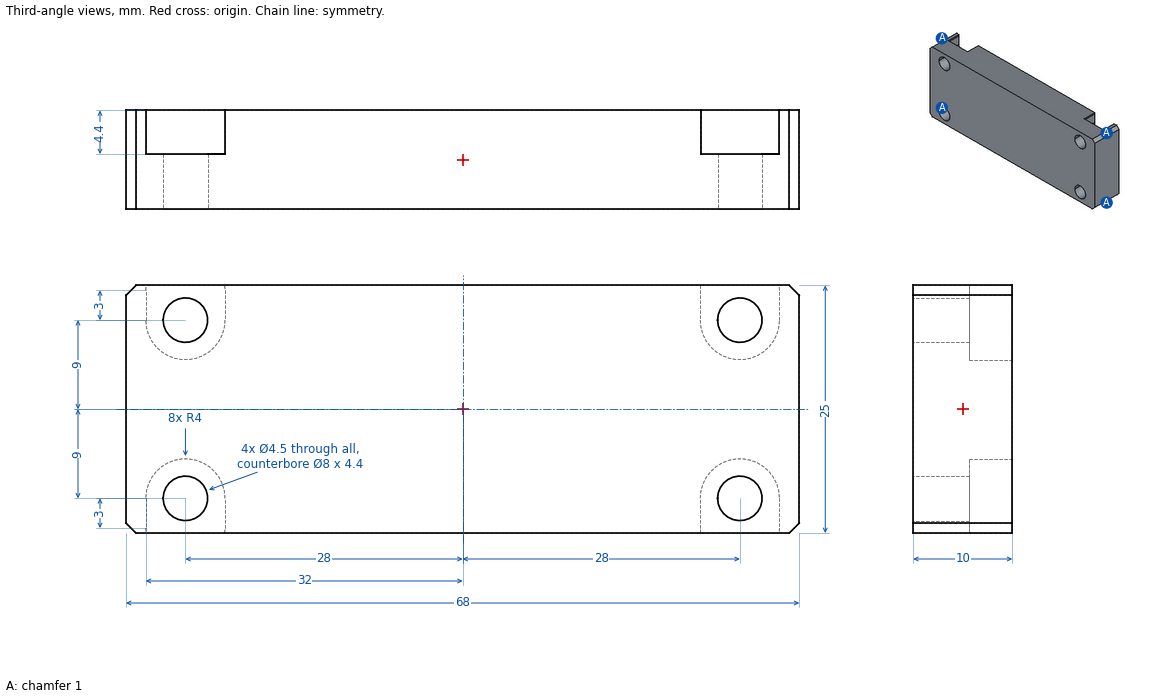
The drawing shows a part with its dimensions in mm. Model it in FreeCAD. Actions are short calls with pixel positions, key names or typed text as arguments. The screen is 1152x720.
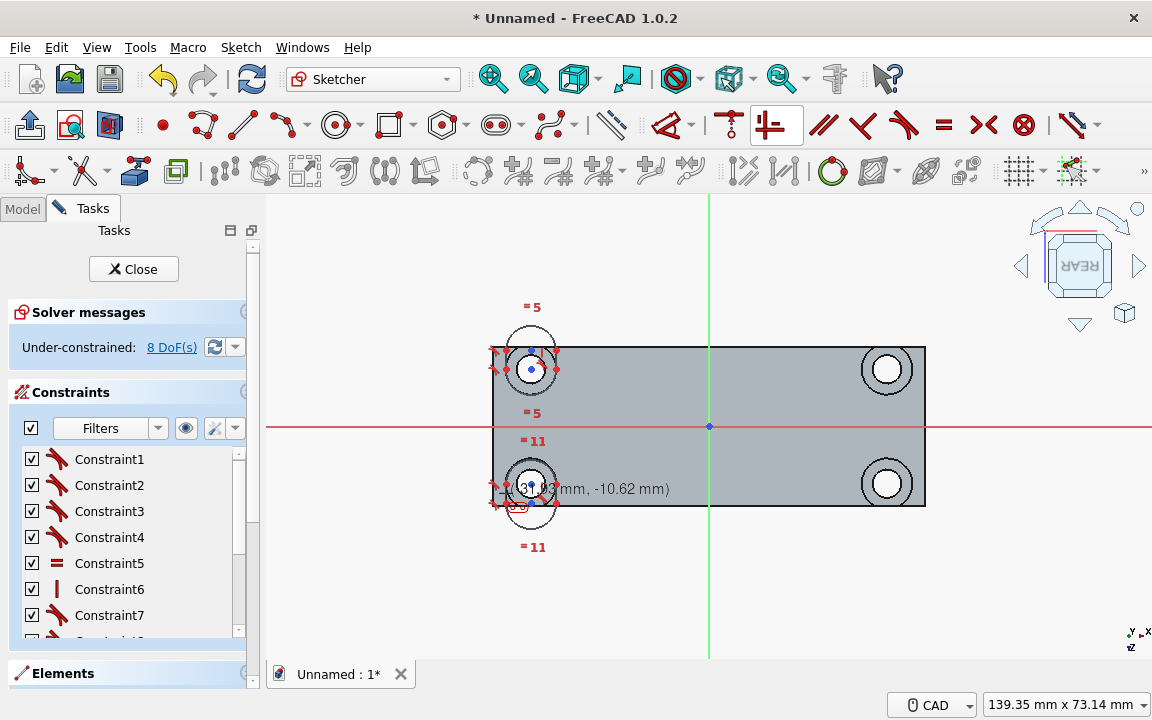
click(887, 369)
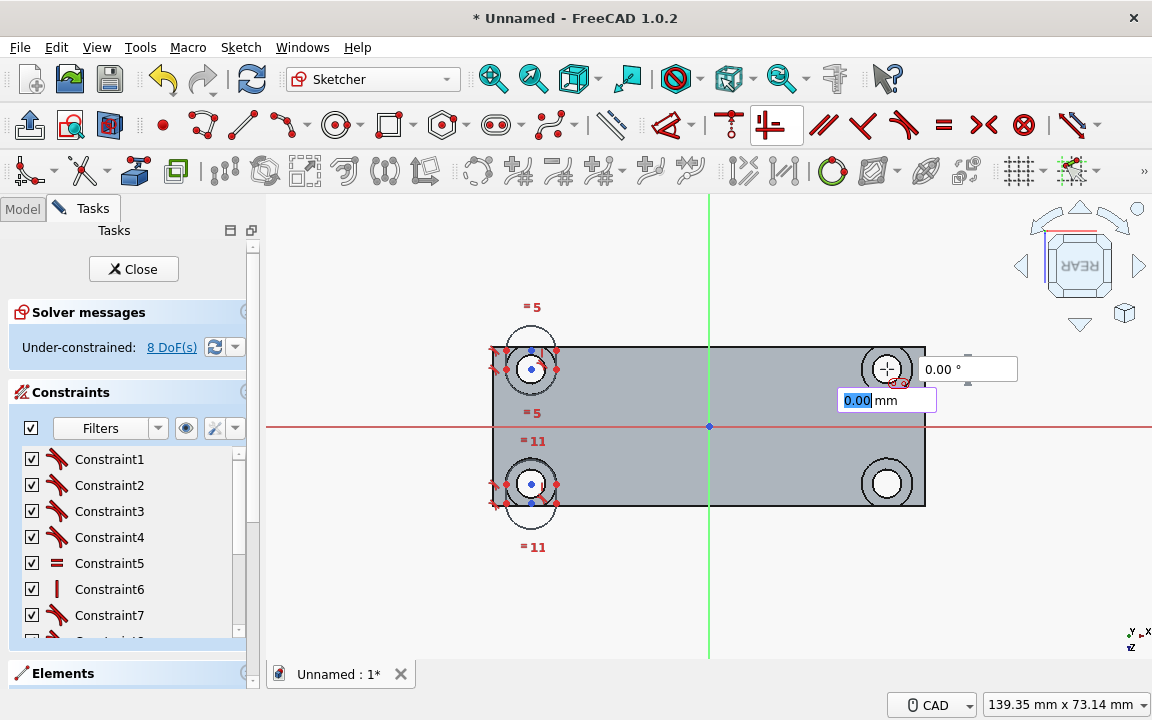
click(887, 350)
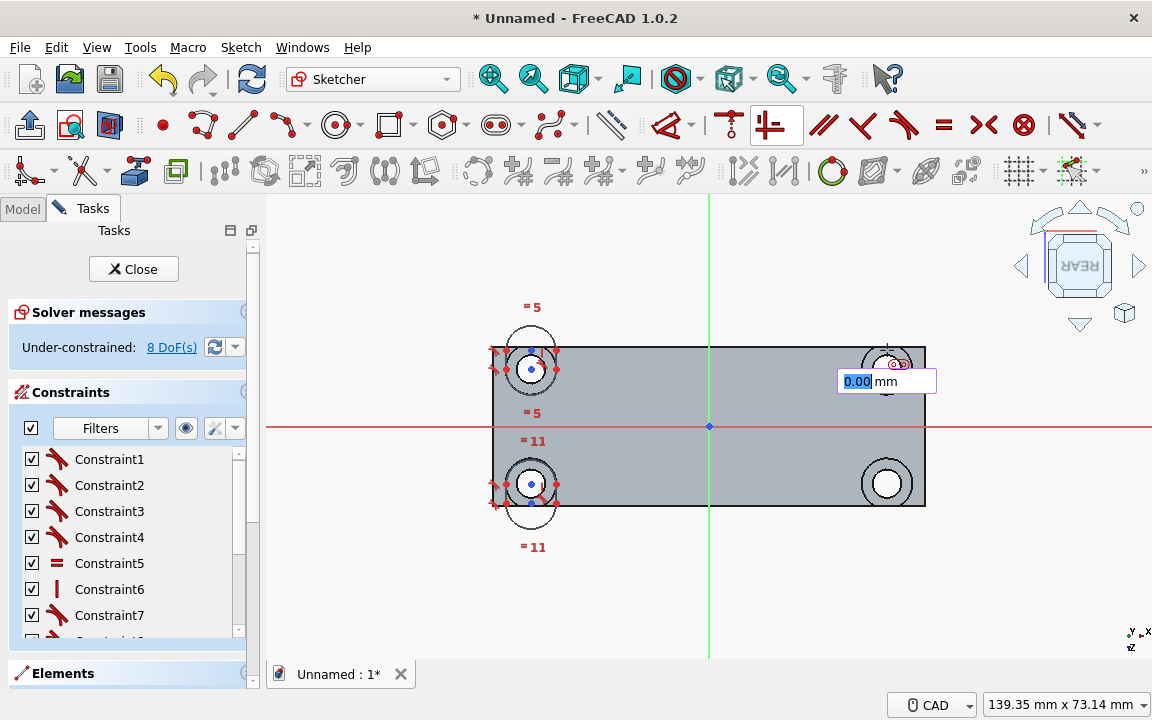
click(912, 360)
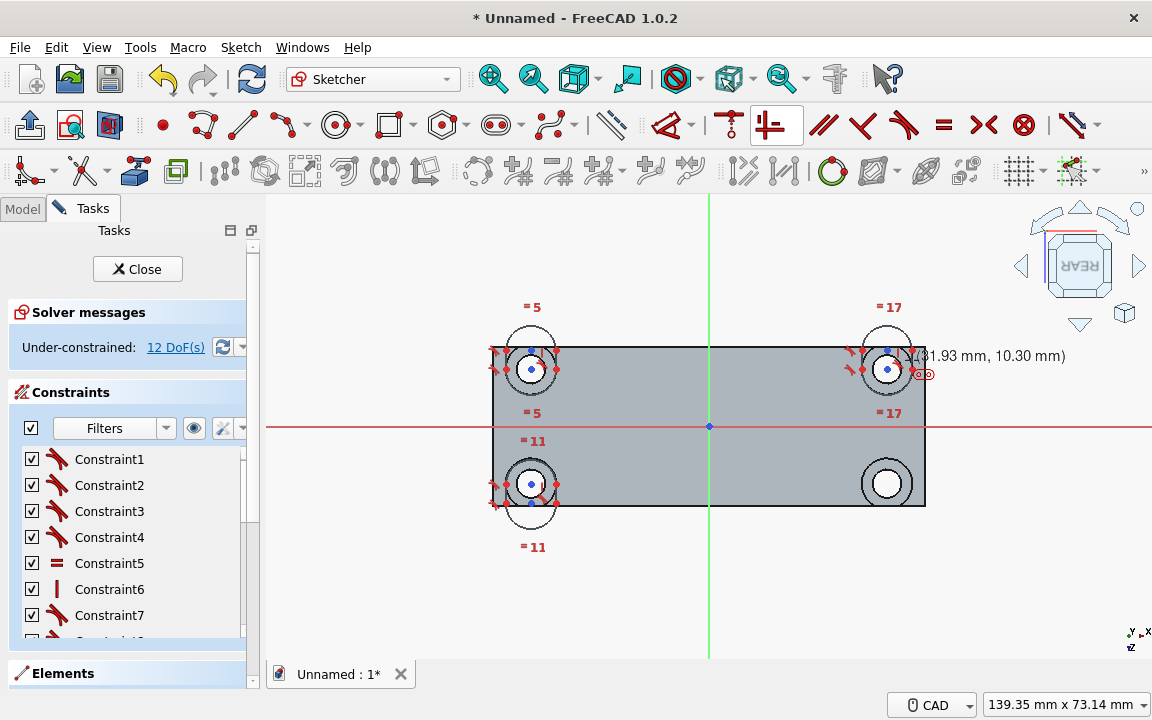
click(887, 503)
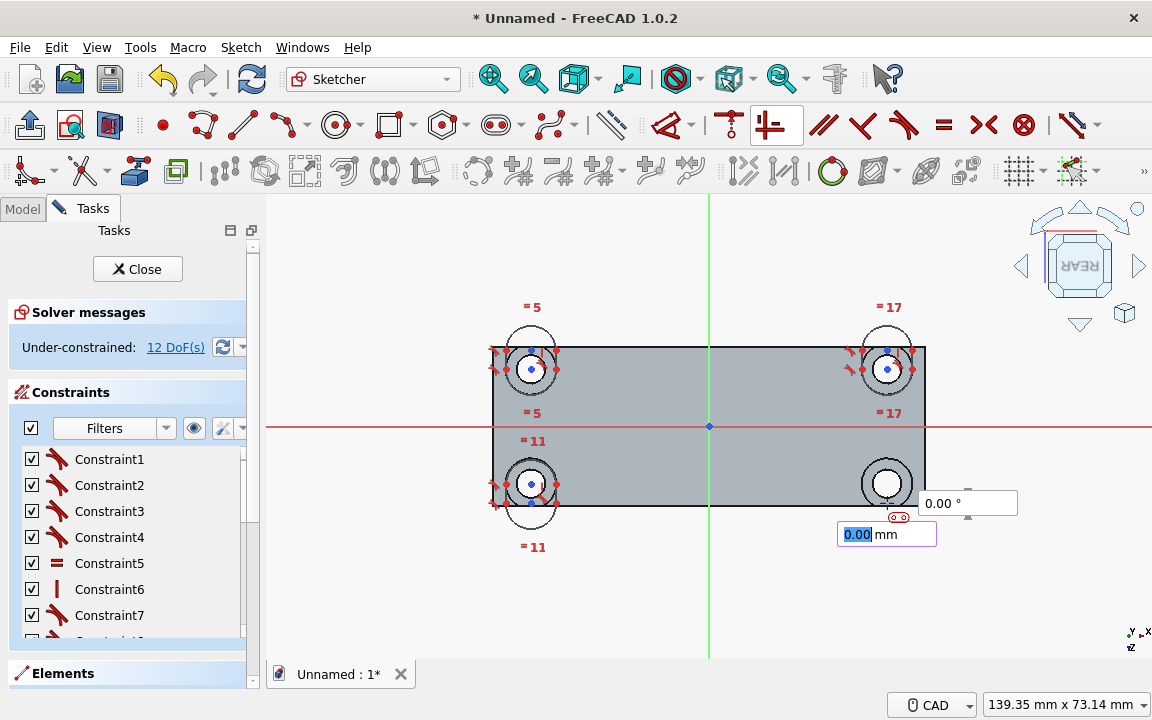
click(887, 484)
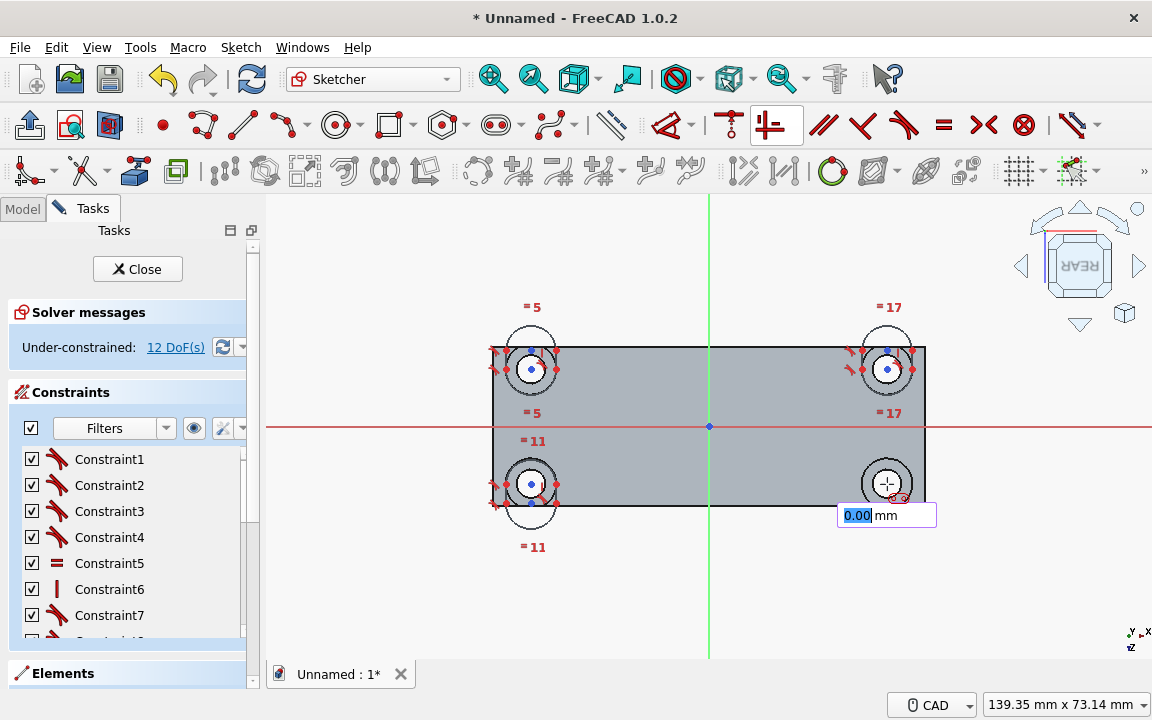
click(912, 493)
key(Escape)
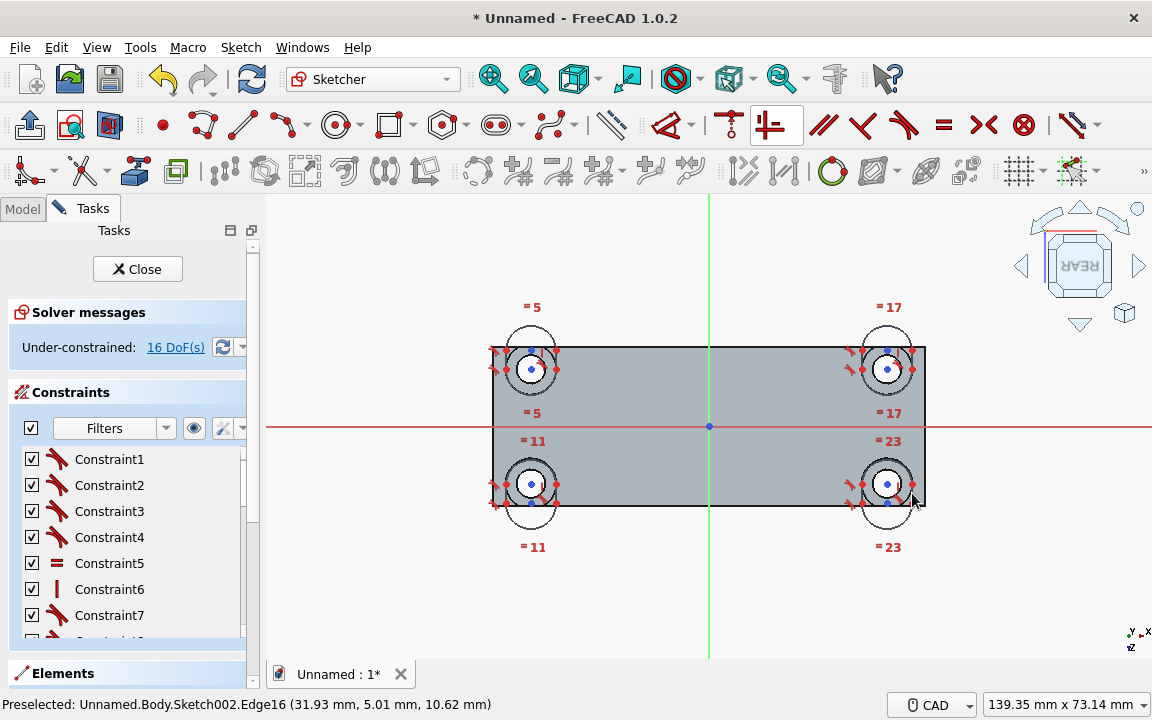
click(516, 390)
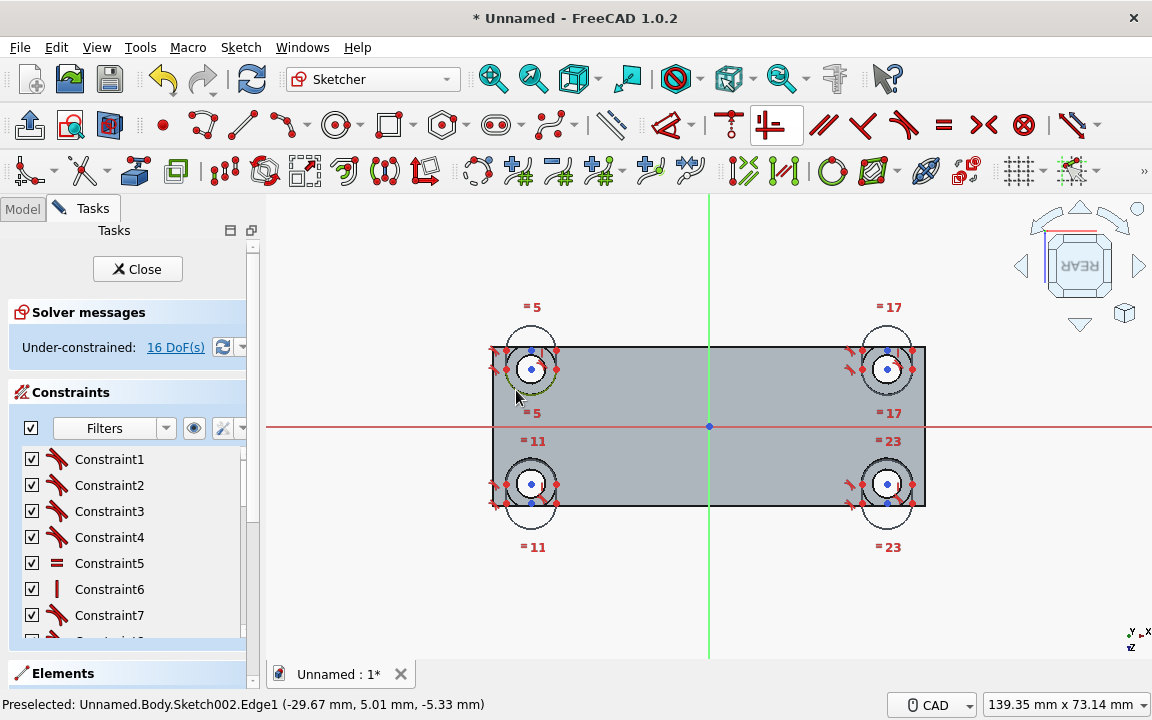
click(516, 524)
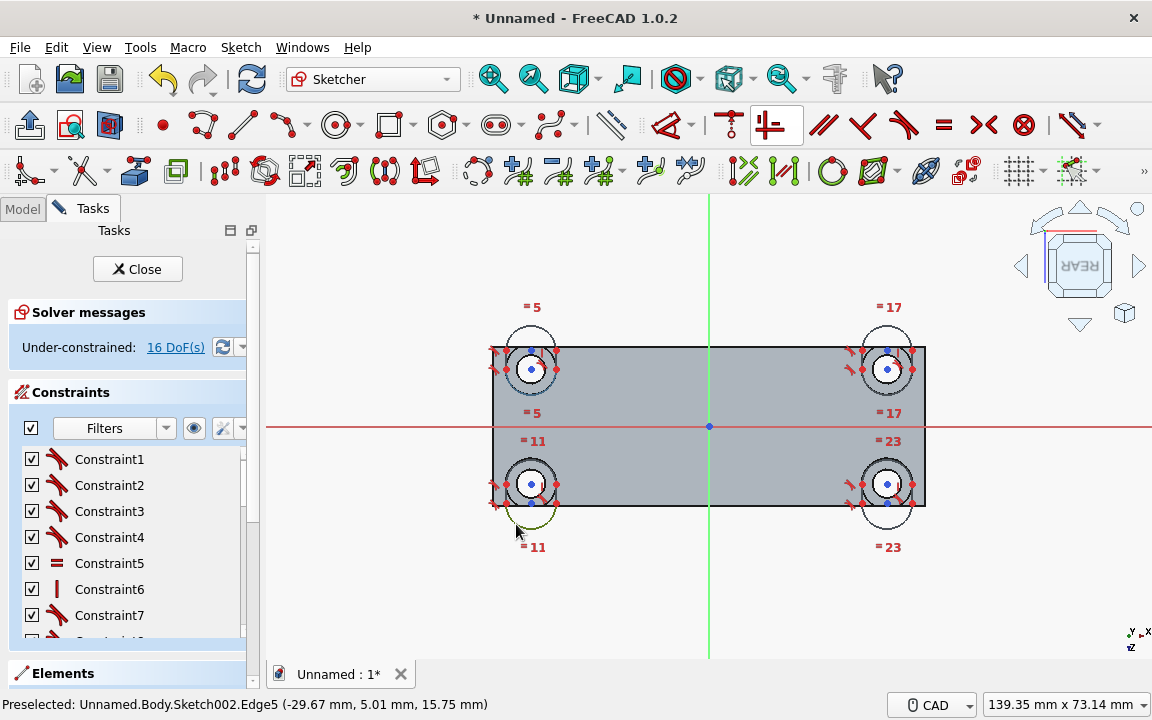
click(872, 390)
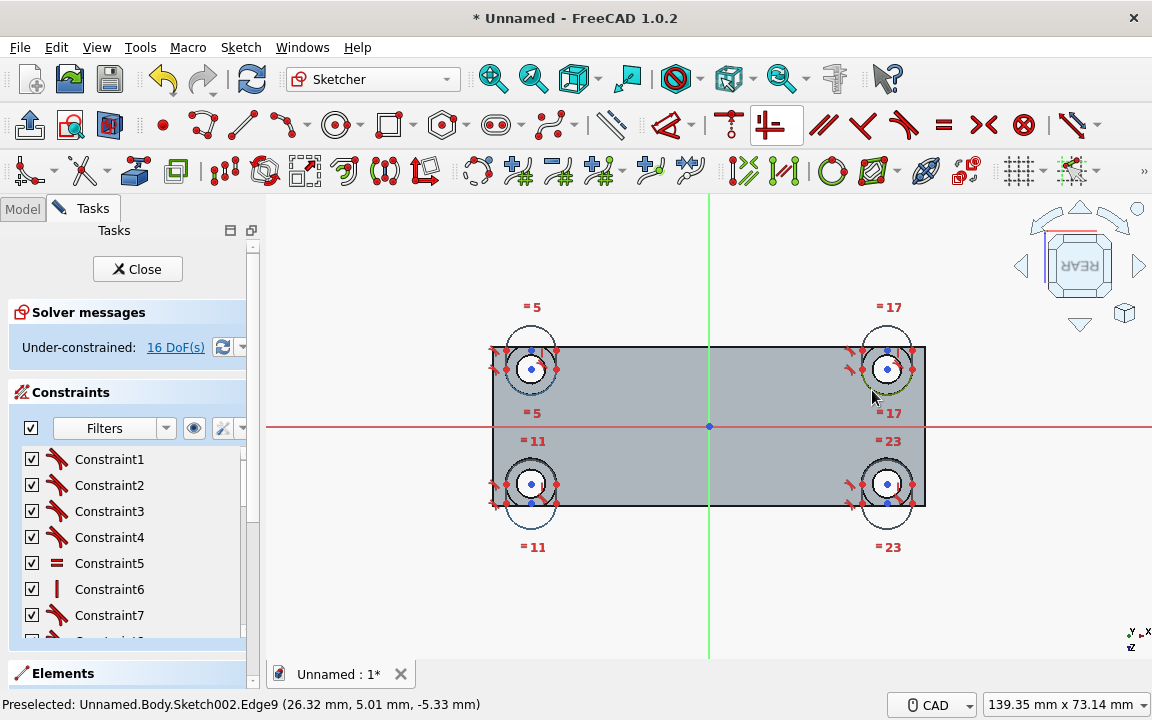
click(872, 524)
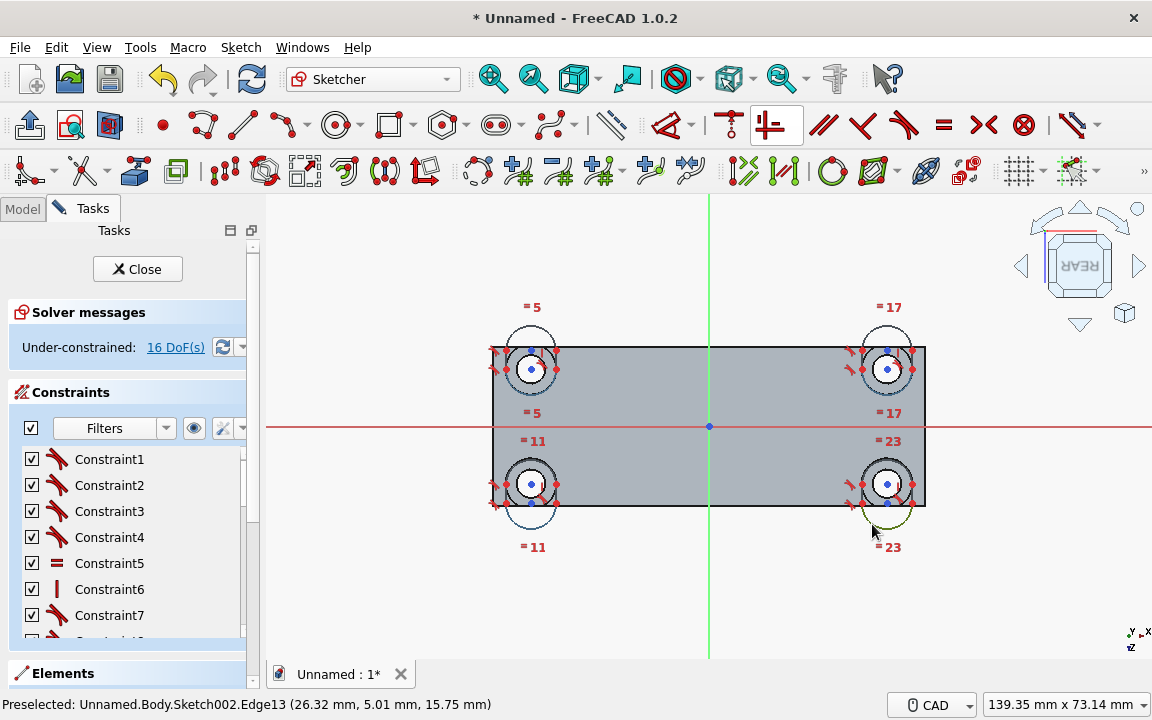
click(944, 126)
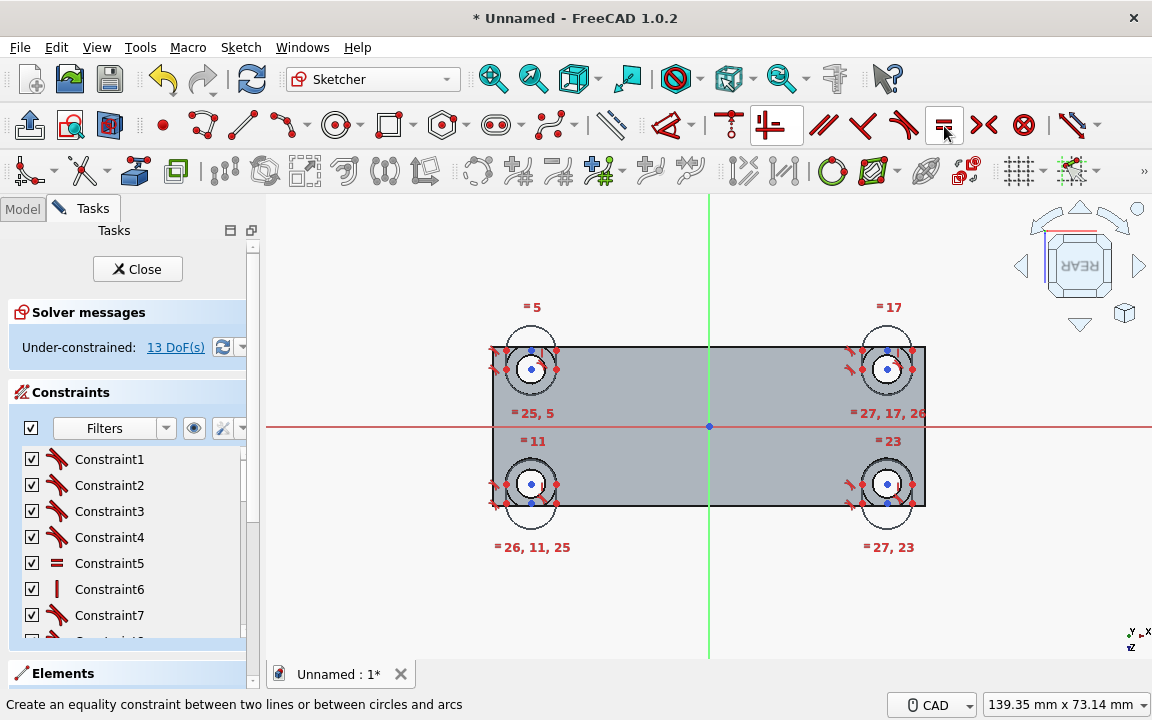
click(531, 351)